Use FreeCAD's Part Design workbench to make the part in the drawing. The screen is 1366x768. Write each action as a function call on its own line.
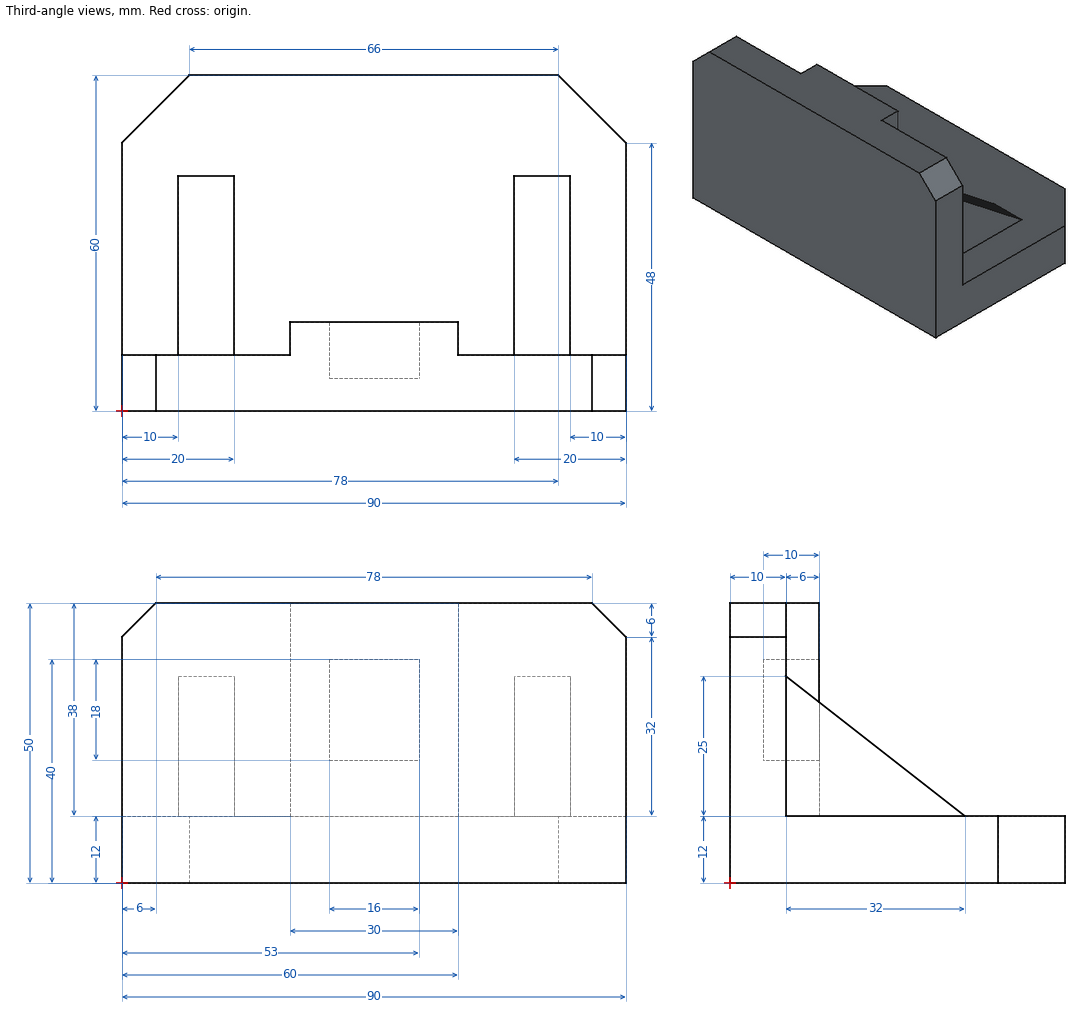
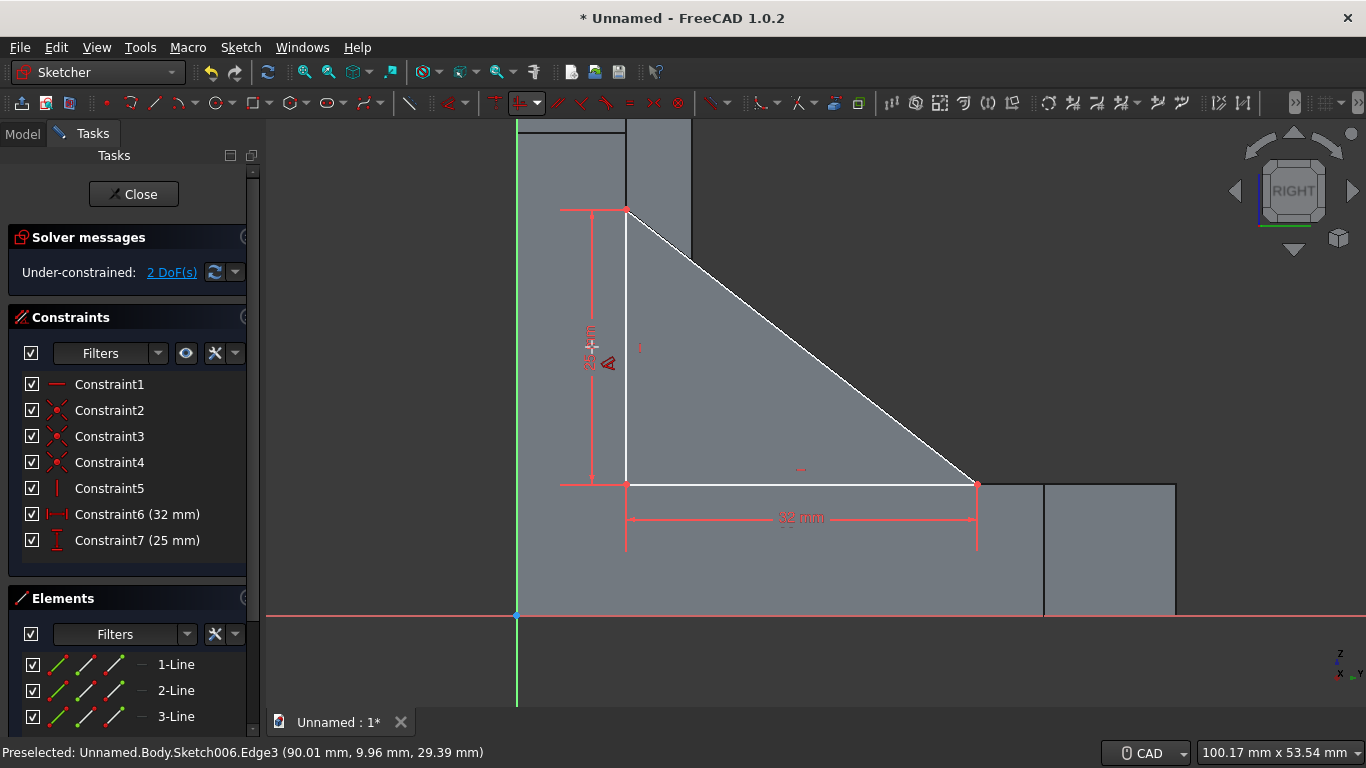
click(626, 485)
click(571, 650)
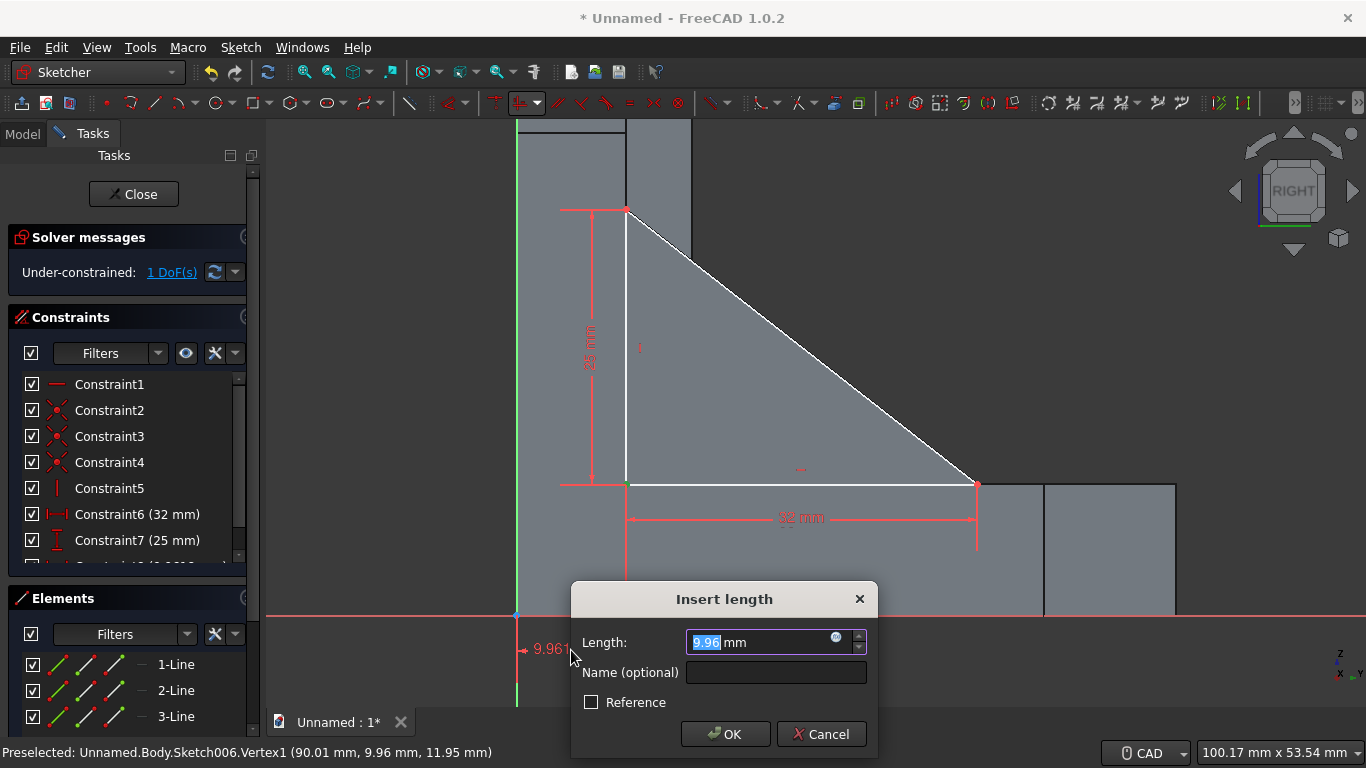
text(10)
key(Return)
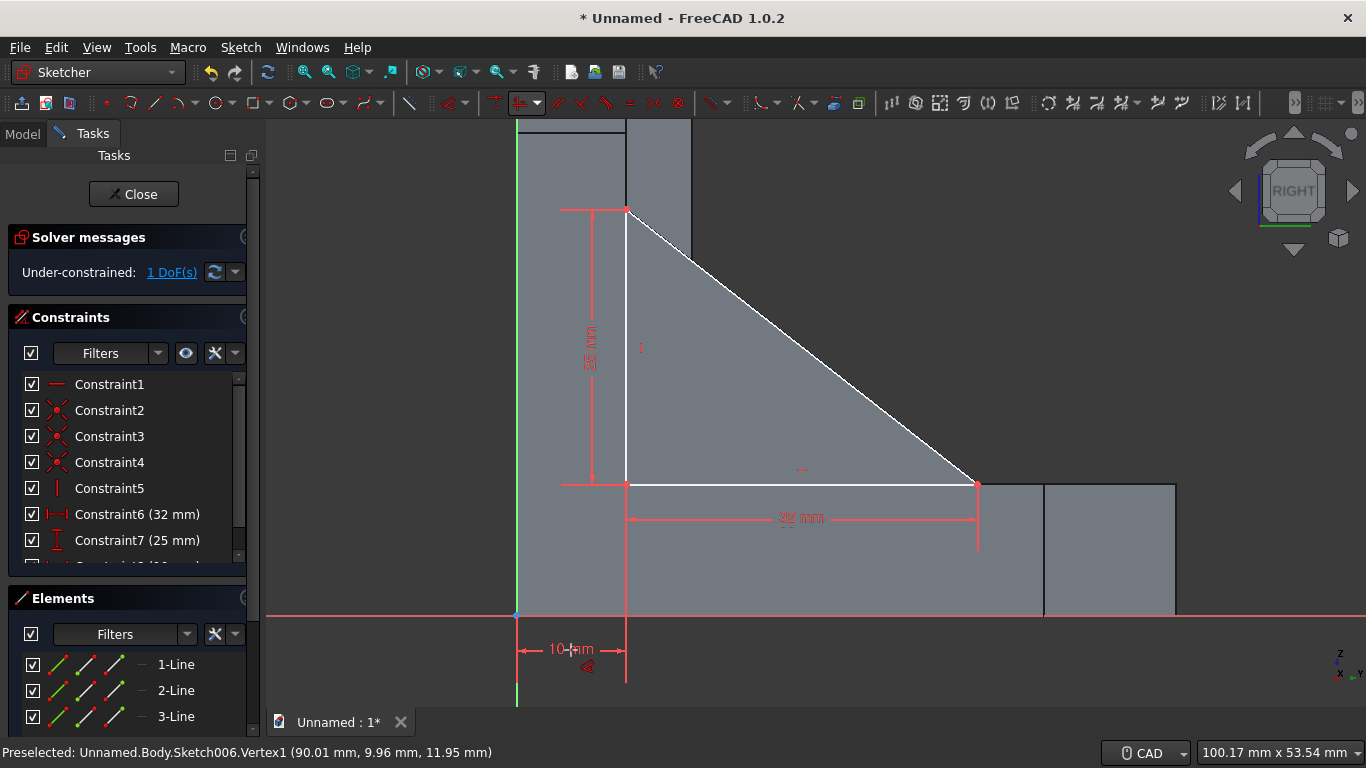
click(626, 485)
click(483, 550)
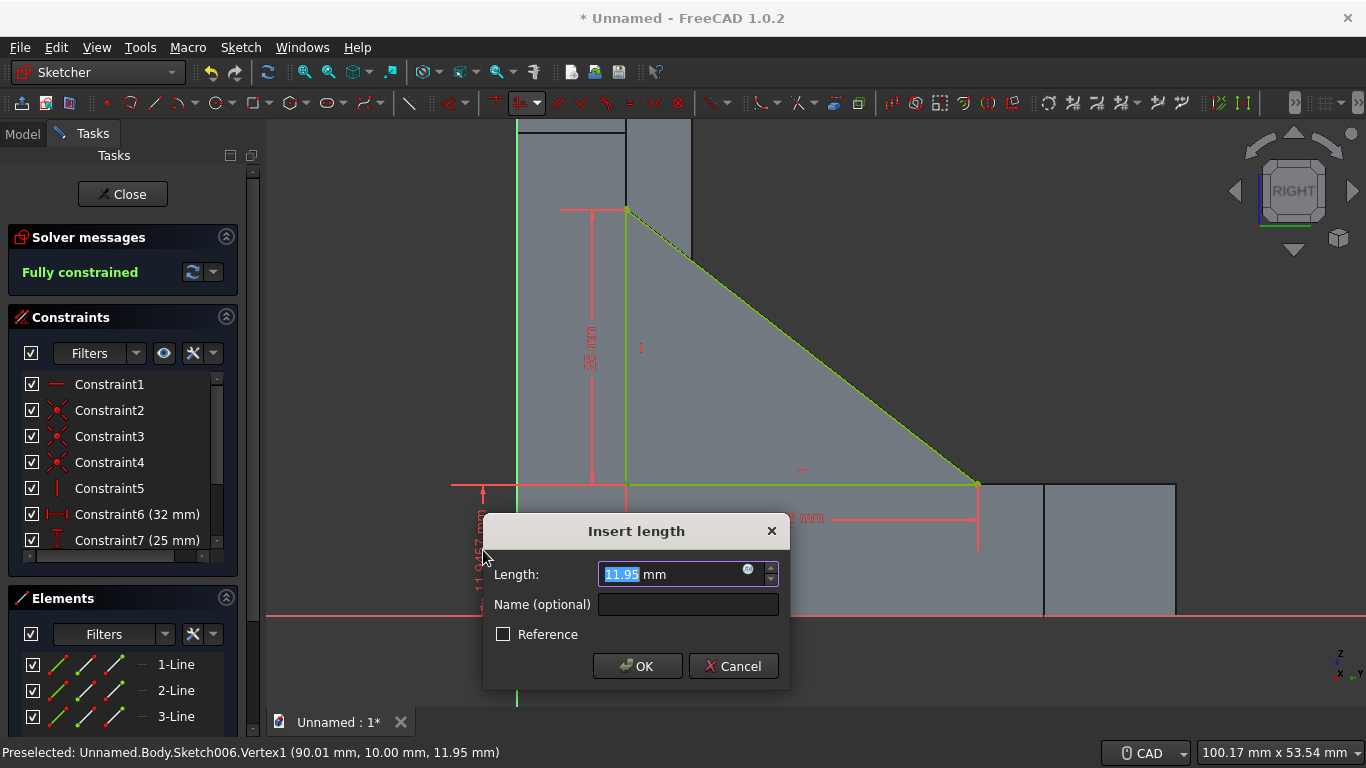
text(12)
key(Return)
key(Escape)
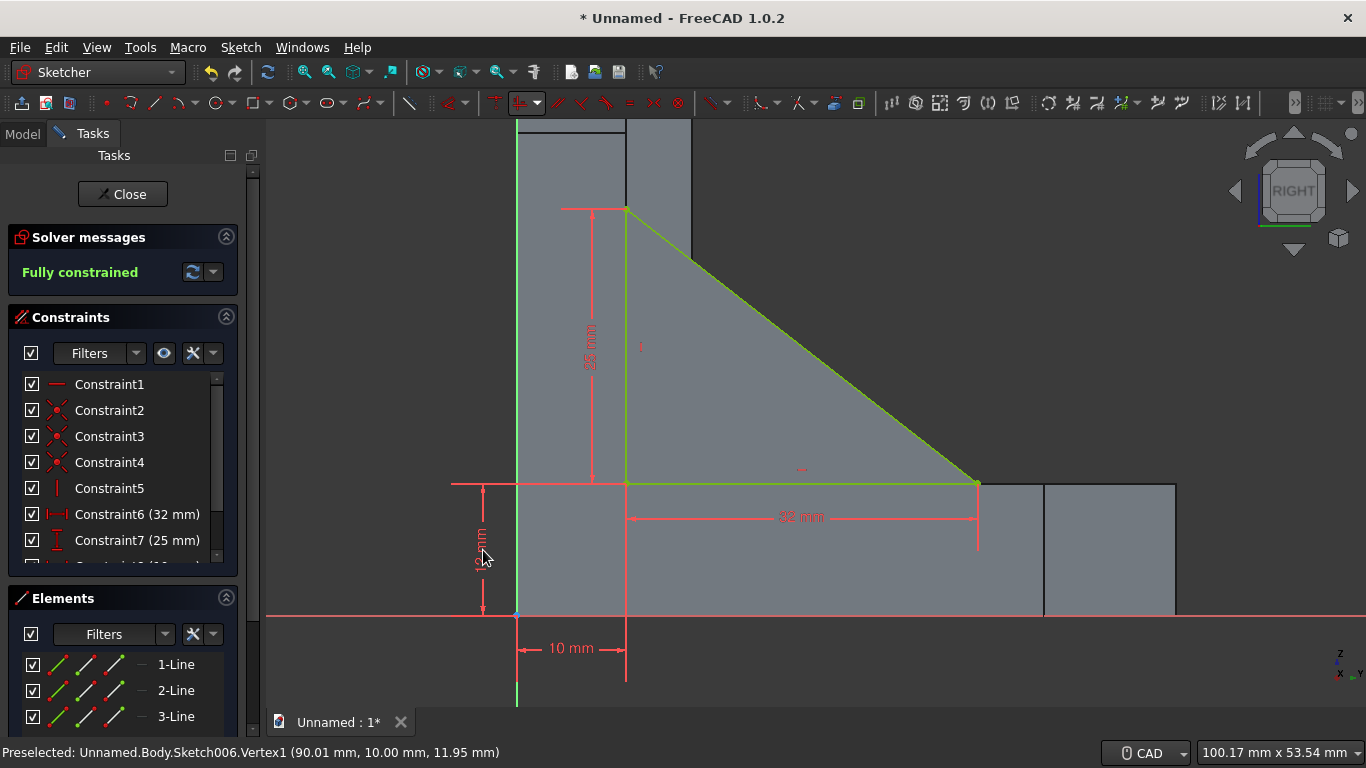
click(123, 194)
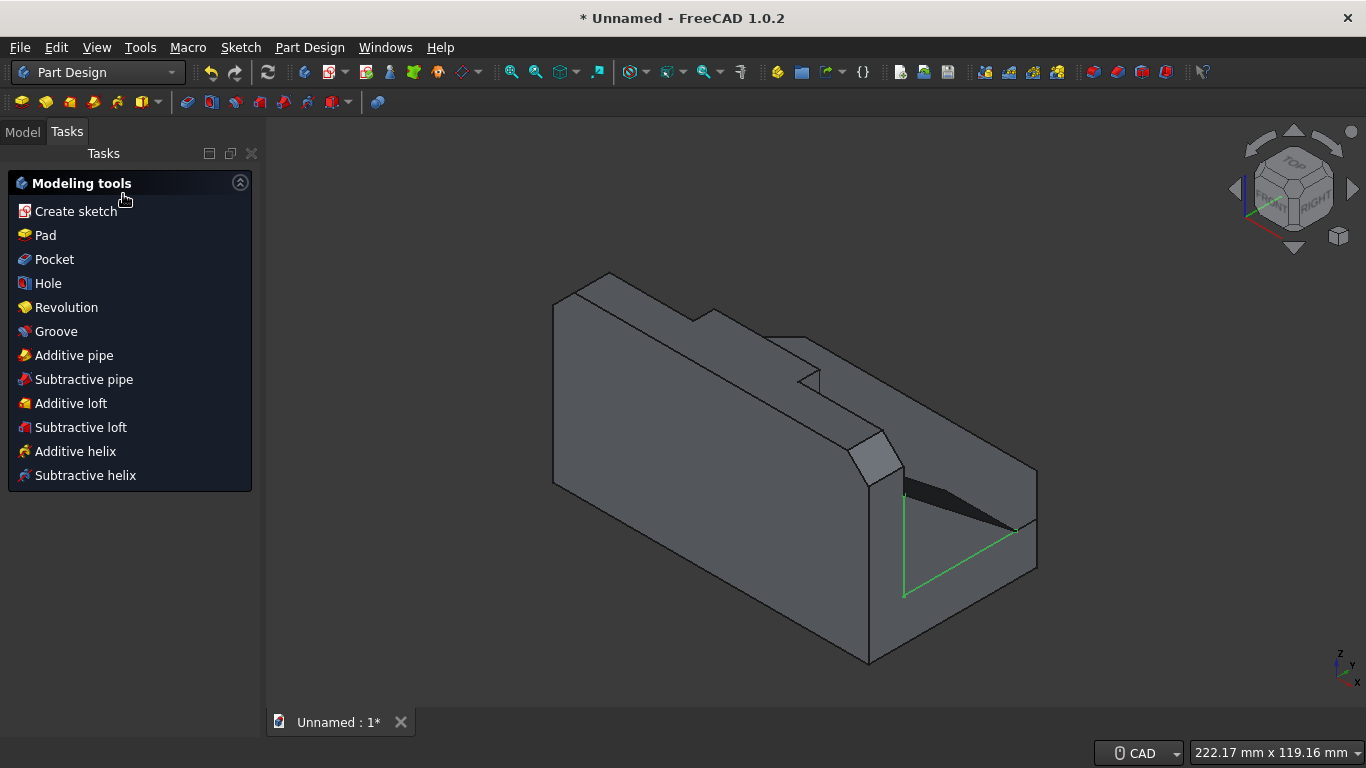
click(188, 102)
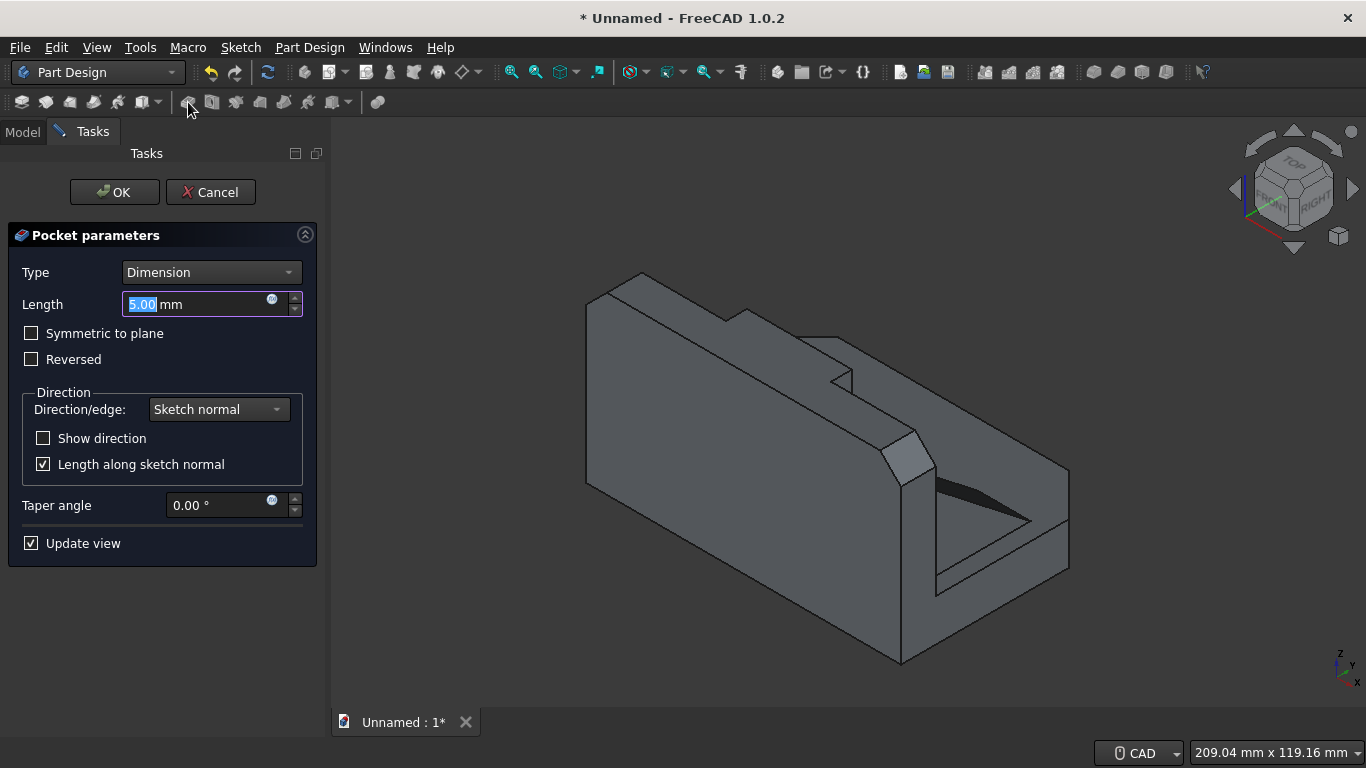
text(10)
key(Tab)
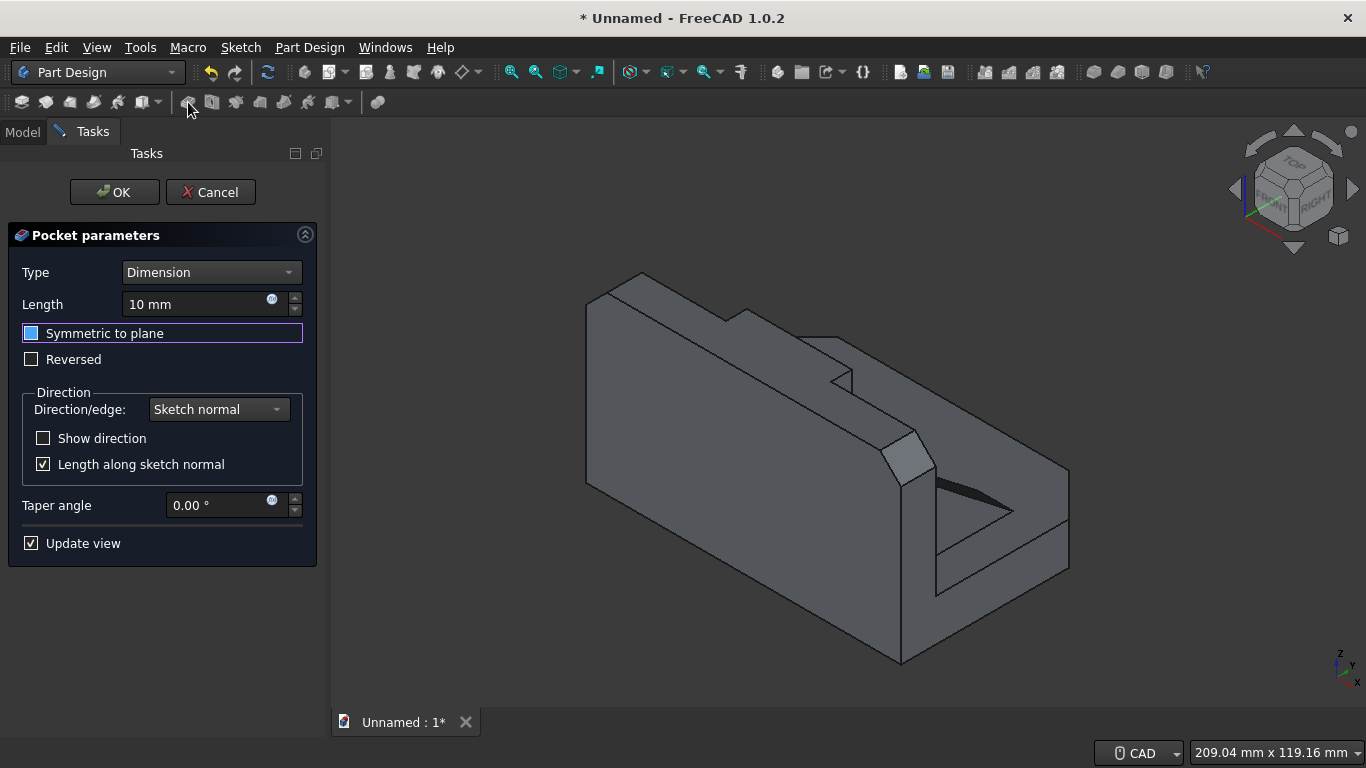
click(115, 192)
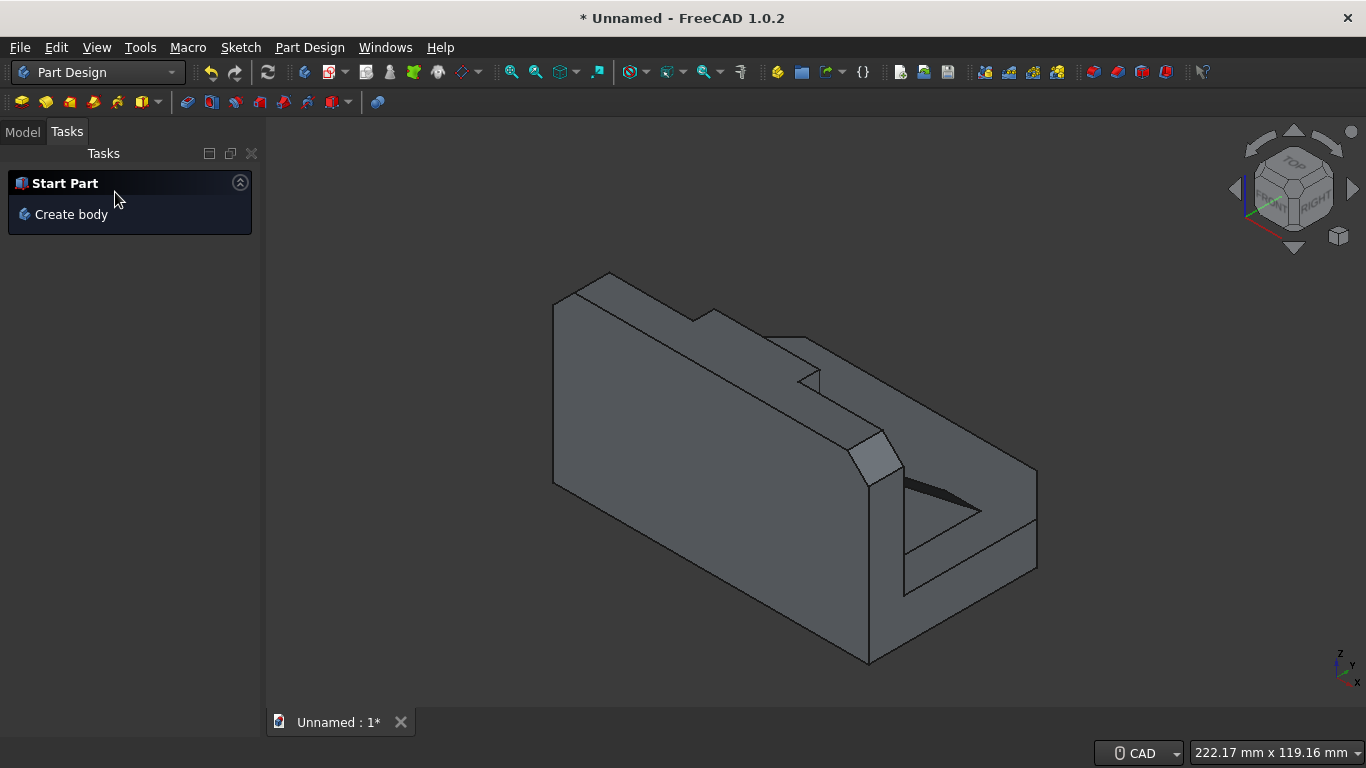
key(6)